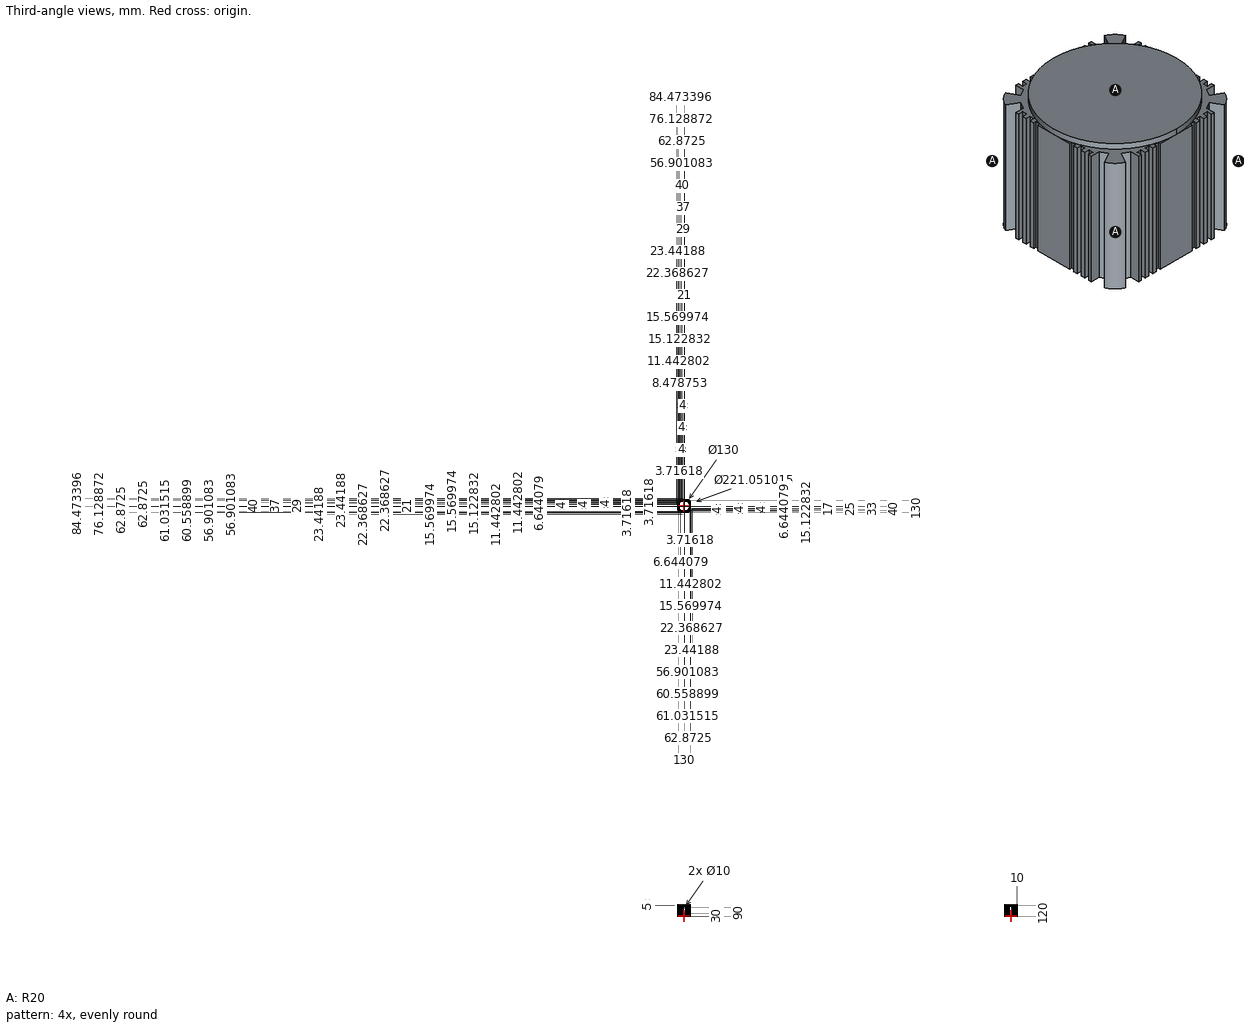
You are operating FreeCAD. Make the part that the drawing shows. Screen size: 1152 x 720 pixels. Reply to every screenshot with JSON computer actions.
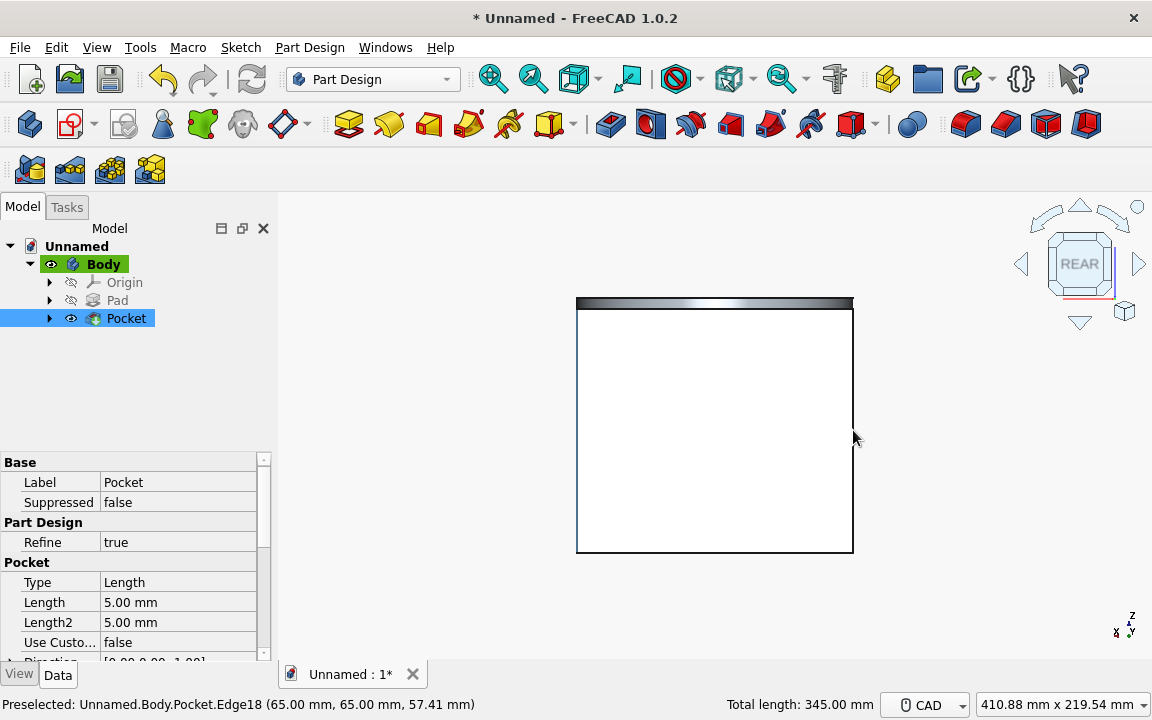
{"action": "left_click", "coordinate": [853, 430], "text": "ctrl"}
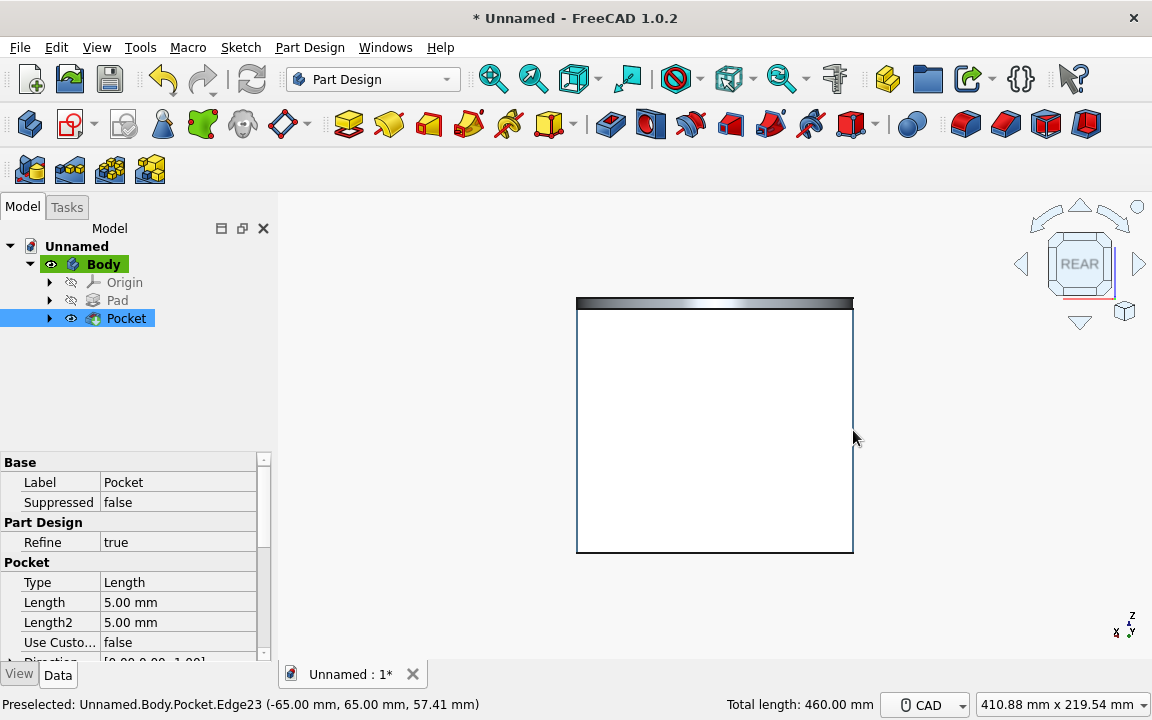
{"action": "left_click", "coordinate": [966, 124]}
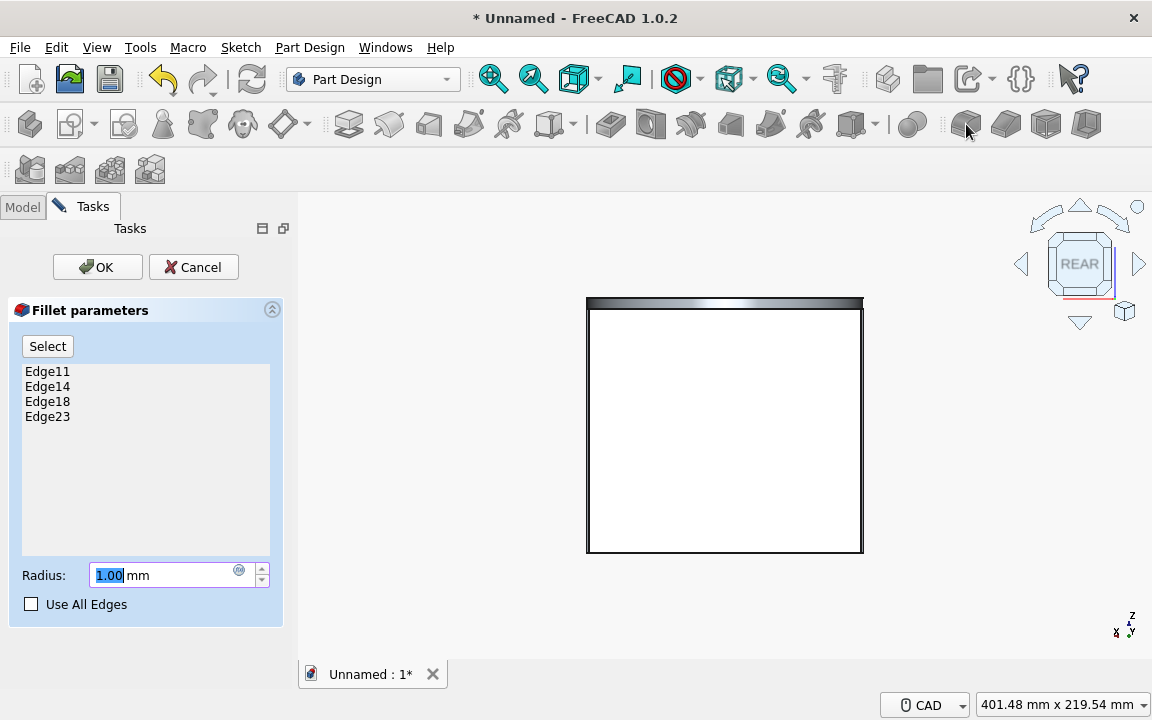
{"action": "type", "text": "20"}
{"action": "key", "text": "Tab"}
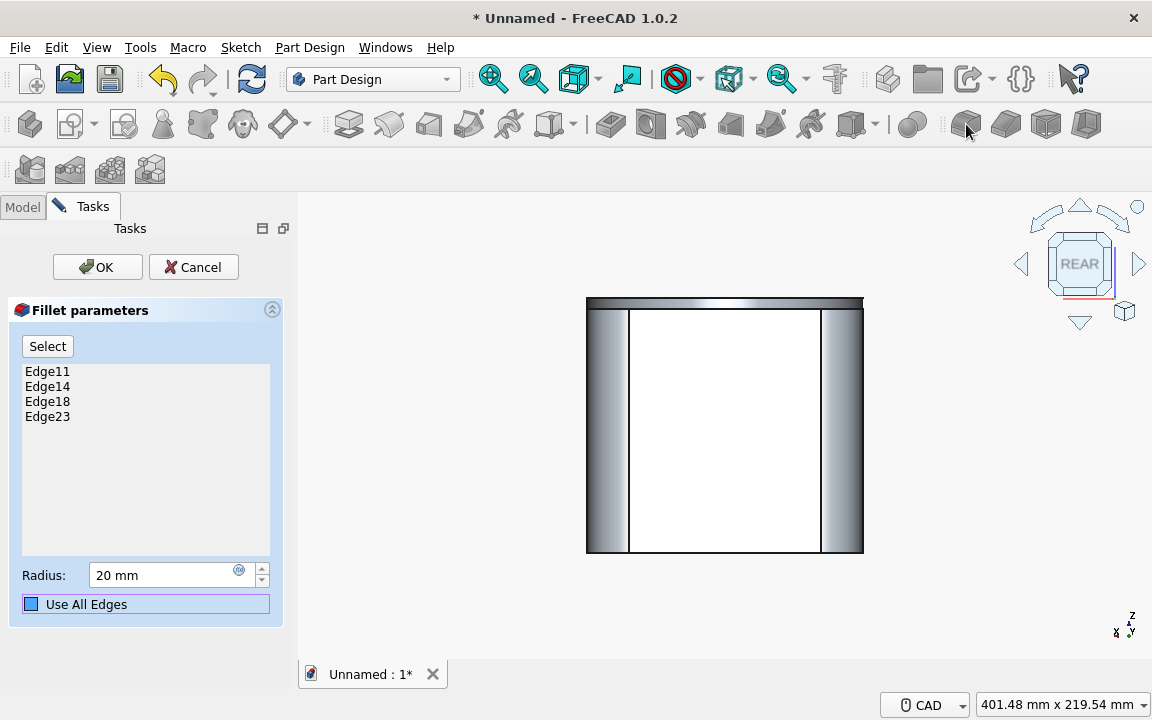
{"action": "left_click", "coordinate": [98, 267]}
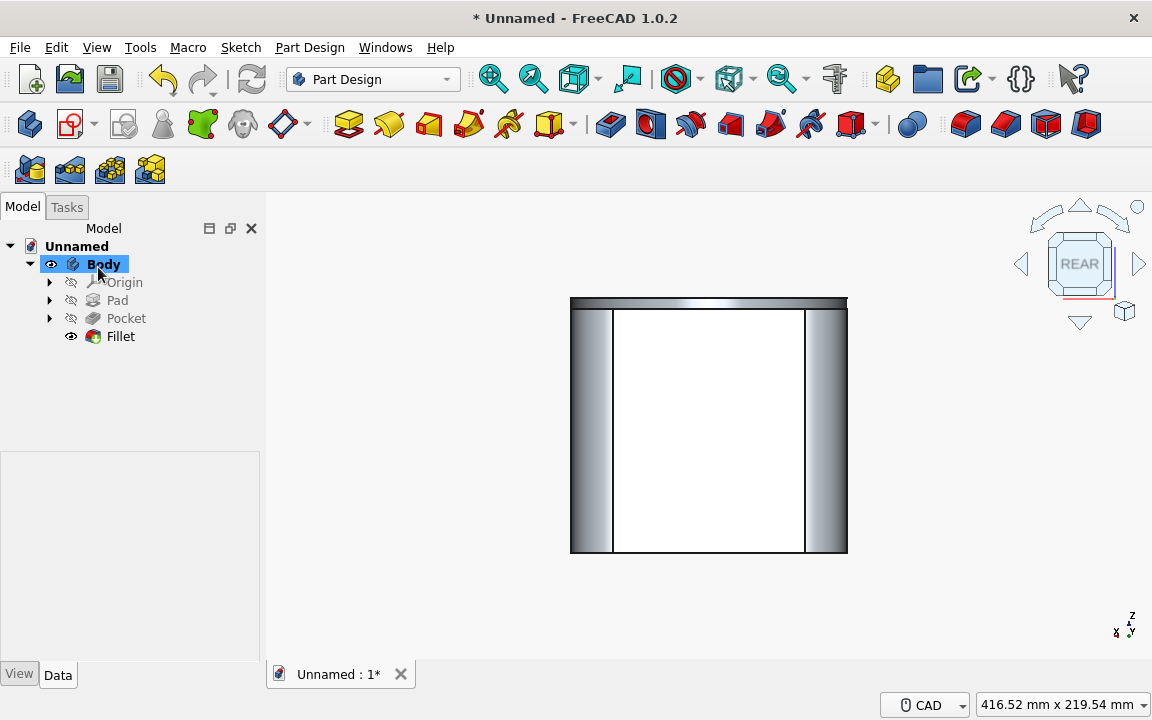
{"action": "key", "text": "0"}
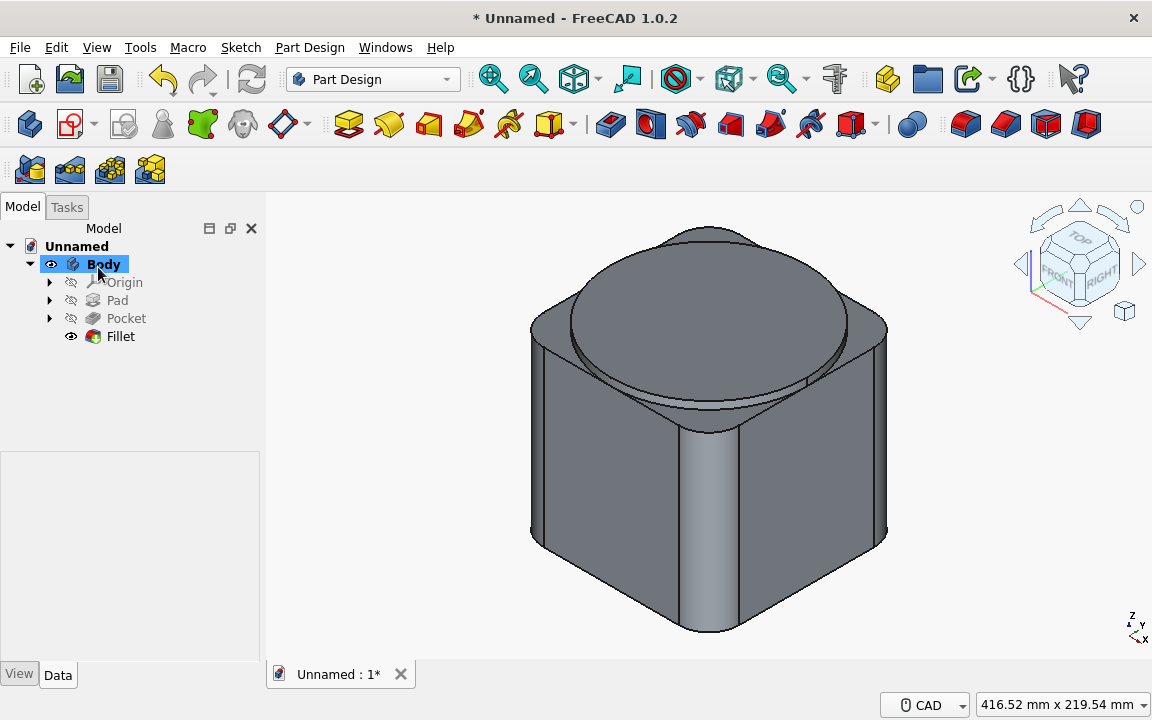
{"action": "left_click", "coordinate": [863, 329]}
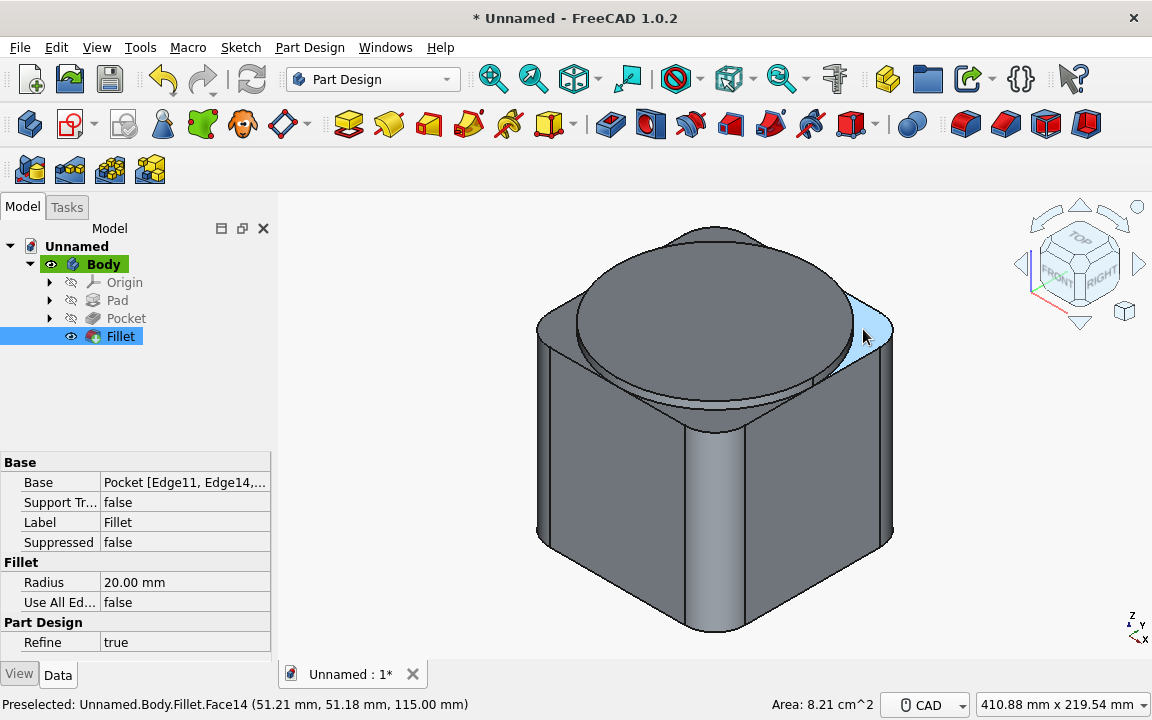
{"action": "left_click", "coordinate": [70, 124]}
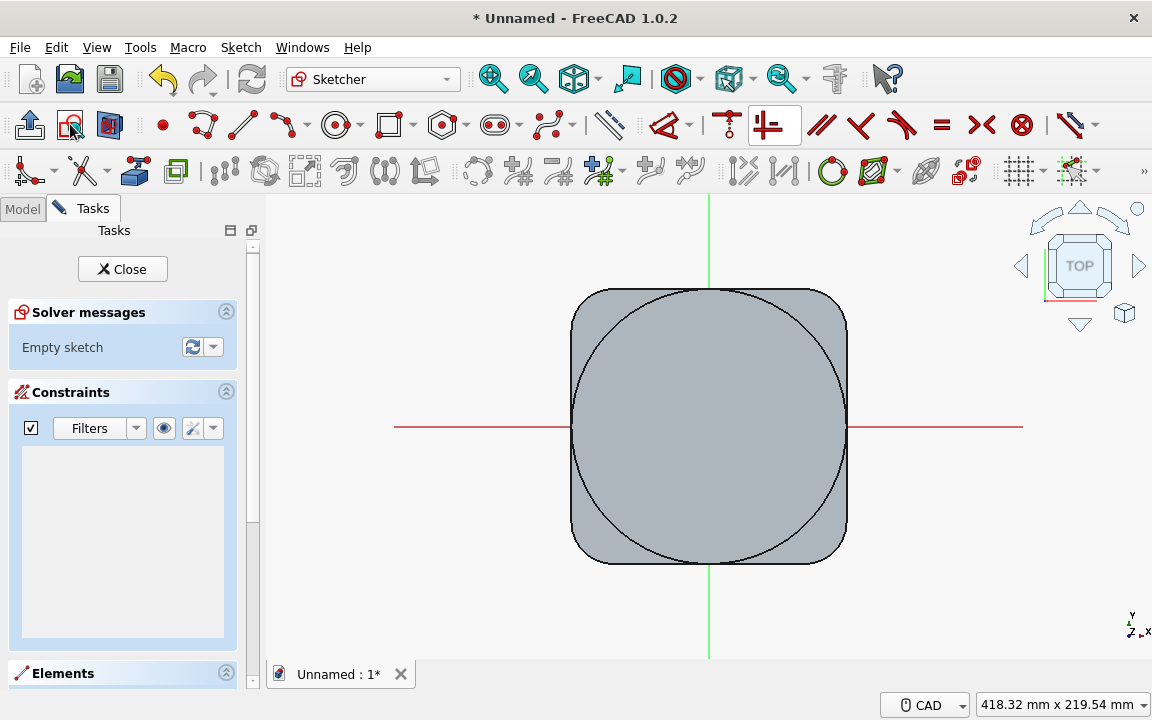
{"action": "left_click", "coordinate": [110, 126]}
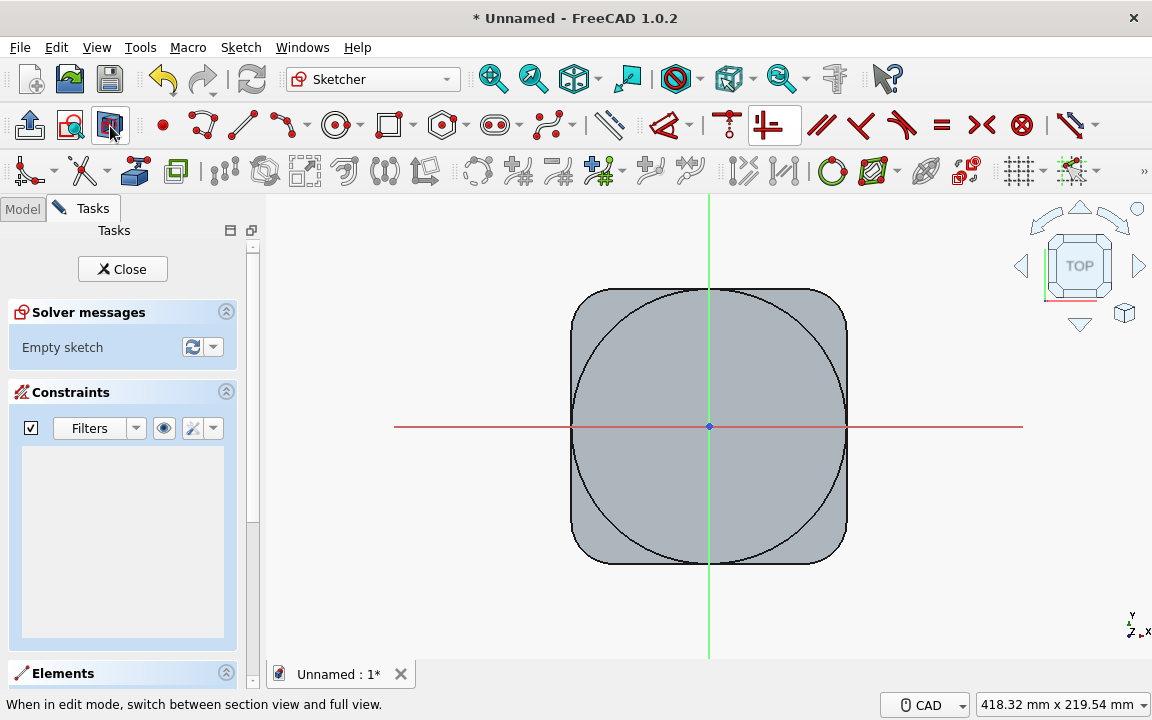
{"action": "scroll", "coordinate": [671, 222], "scroll_direction": "up", "scroll_amount": 2}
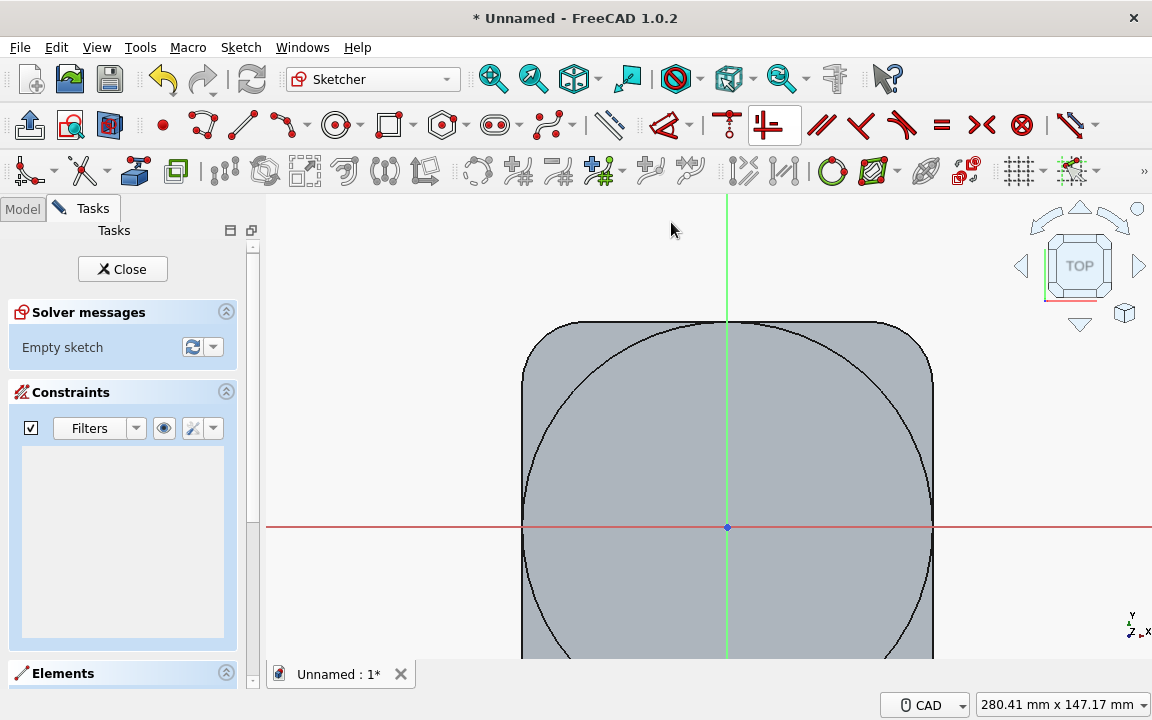
{"action": "left_click", "coordinate": [204, 126]}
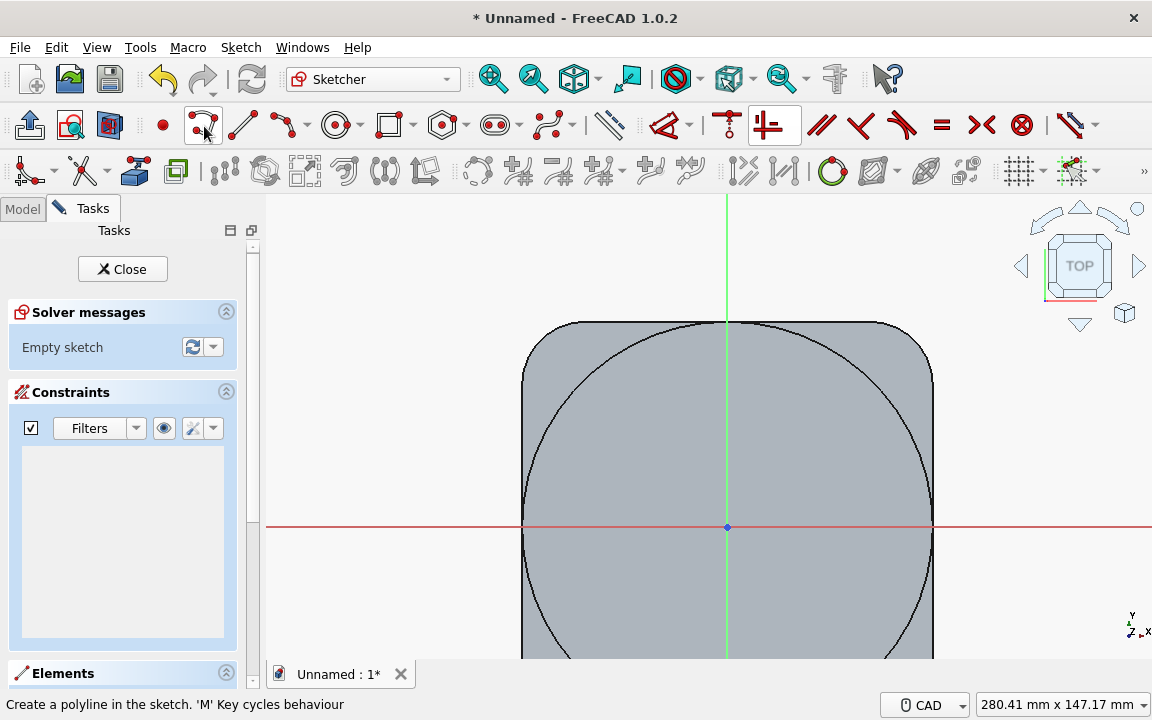
{"action": "left_click", "coordinate": [601, 347]}
{"action": "left_click", "coordinate": [601, 311]}
{"action": "left_click", "coordinate": [553, 311]}
{"action": "left_click", "coordinate": [580, 359]}
{"action": "left_click", "coordinate": [601, 348]}